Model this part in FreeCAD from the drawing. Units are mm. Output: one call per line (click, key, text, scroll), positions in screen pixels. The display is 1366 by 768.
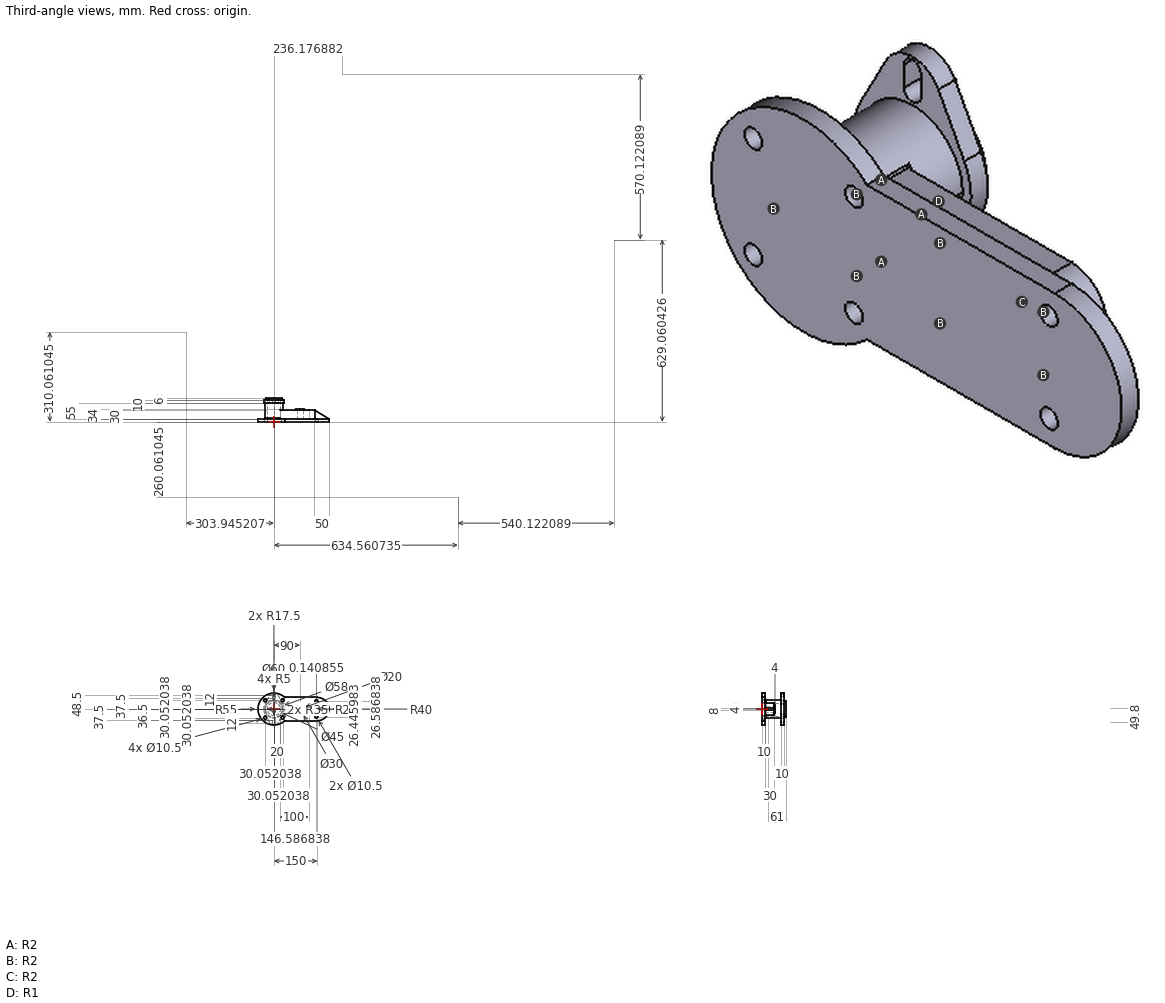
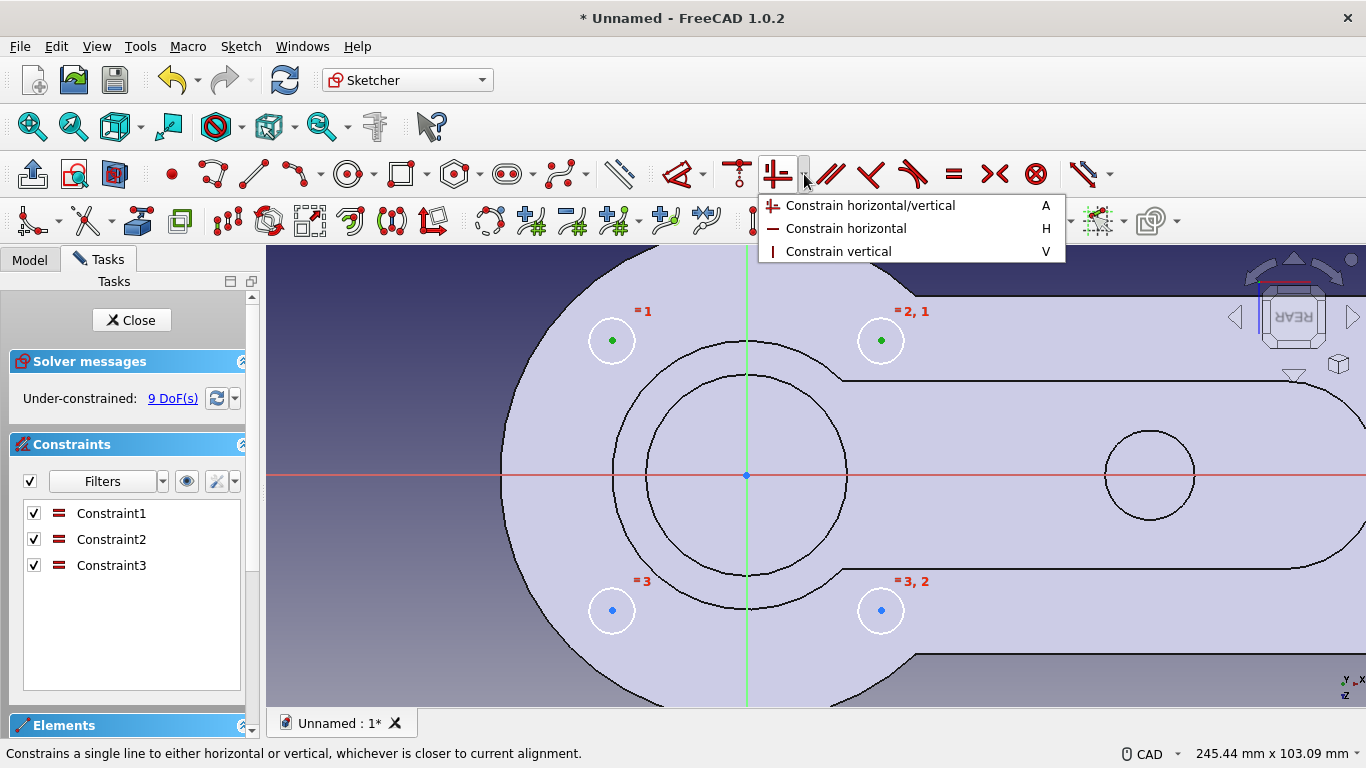
click(912, 228)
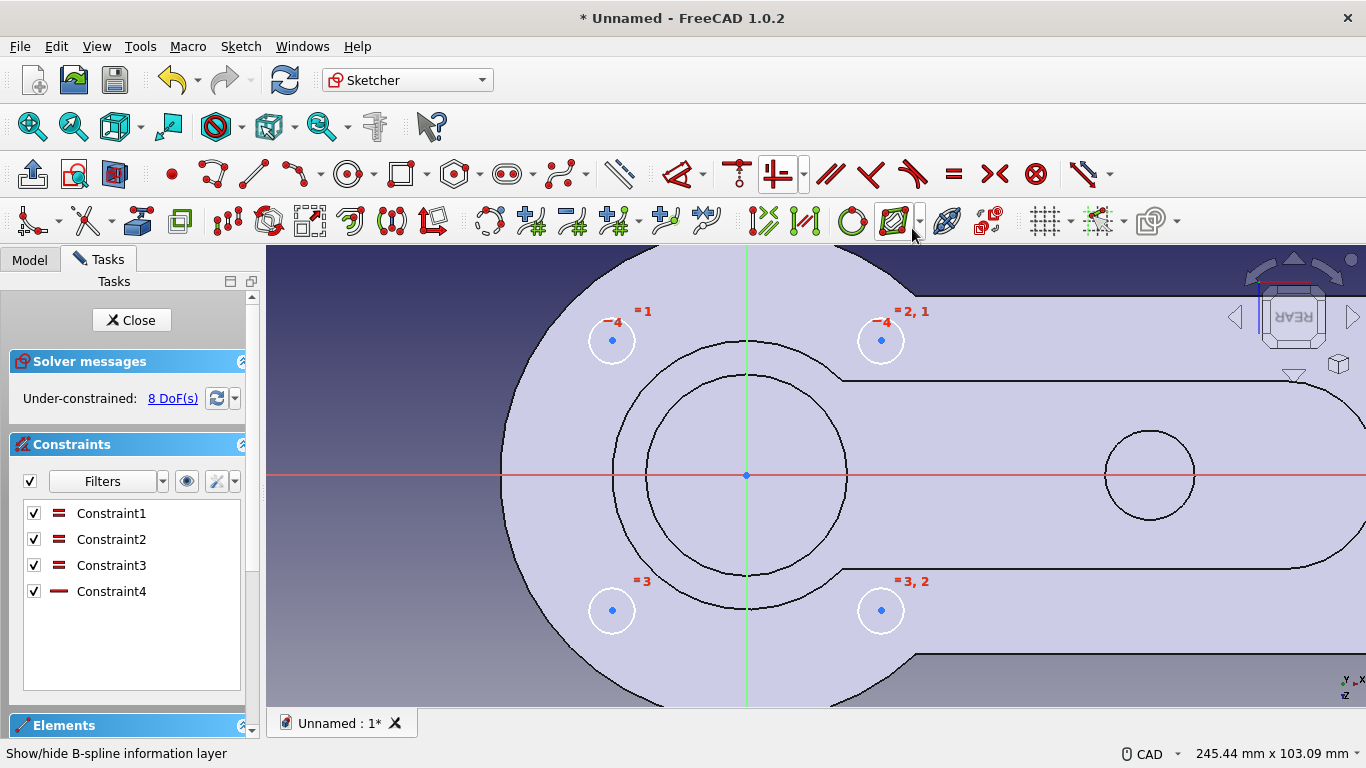
click(881, 341)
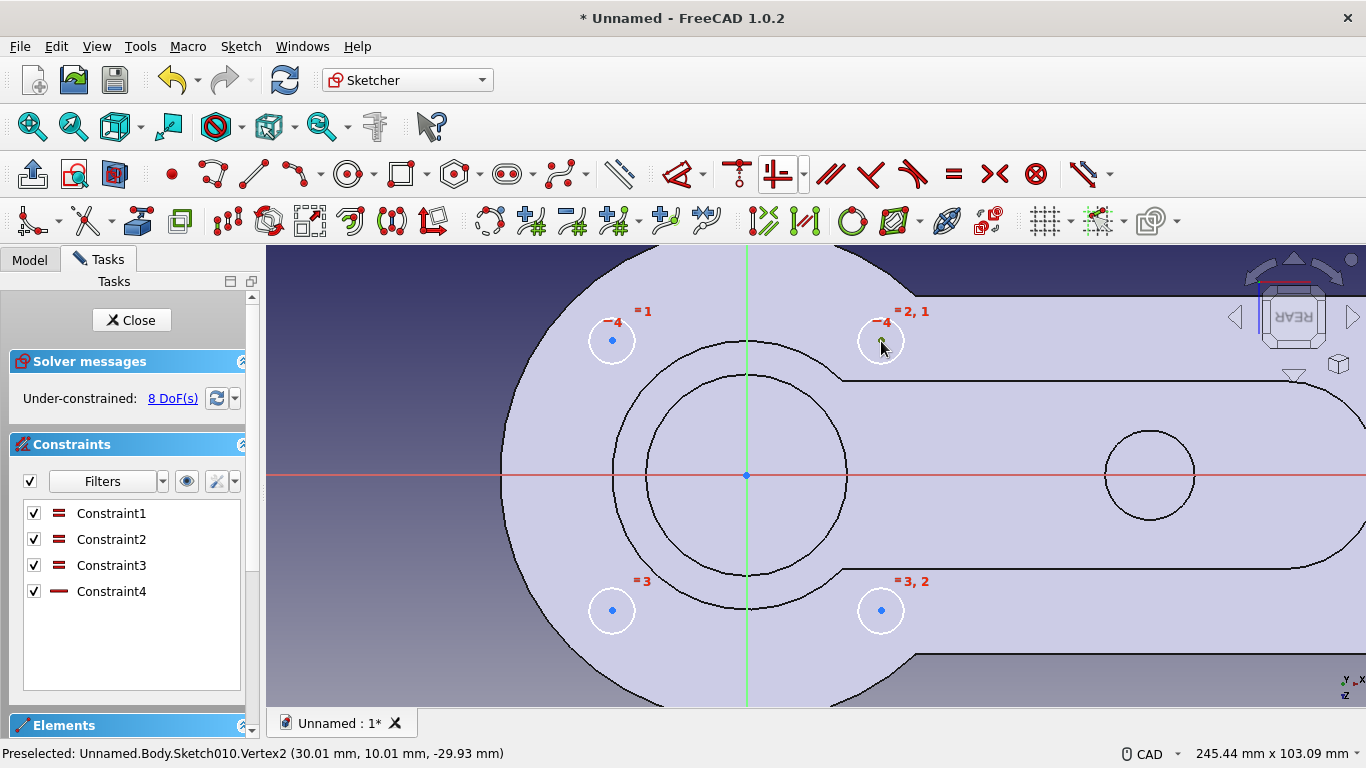
click(881, 611)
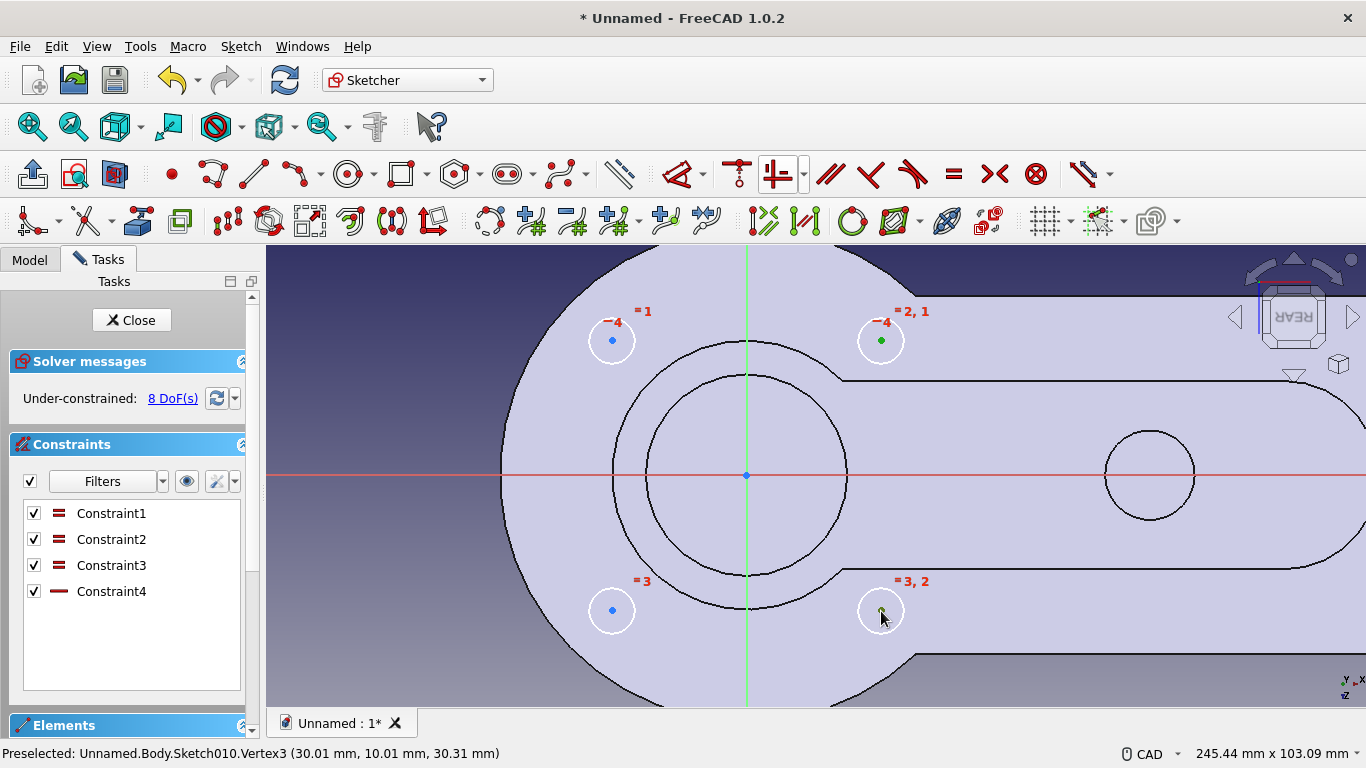
key(v)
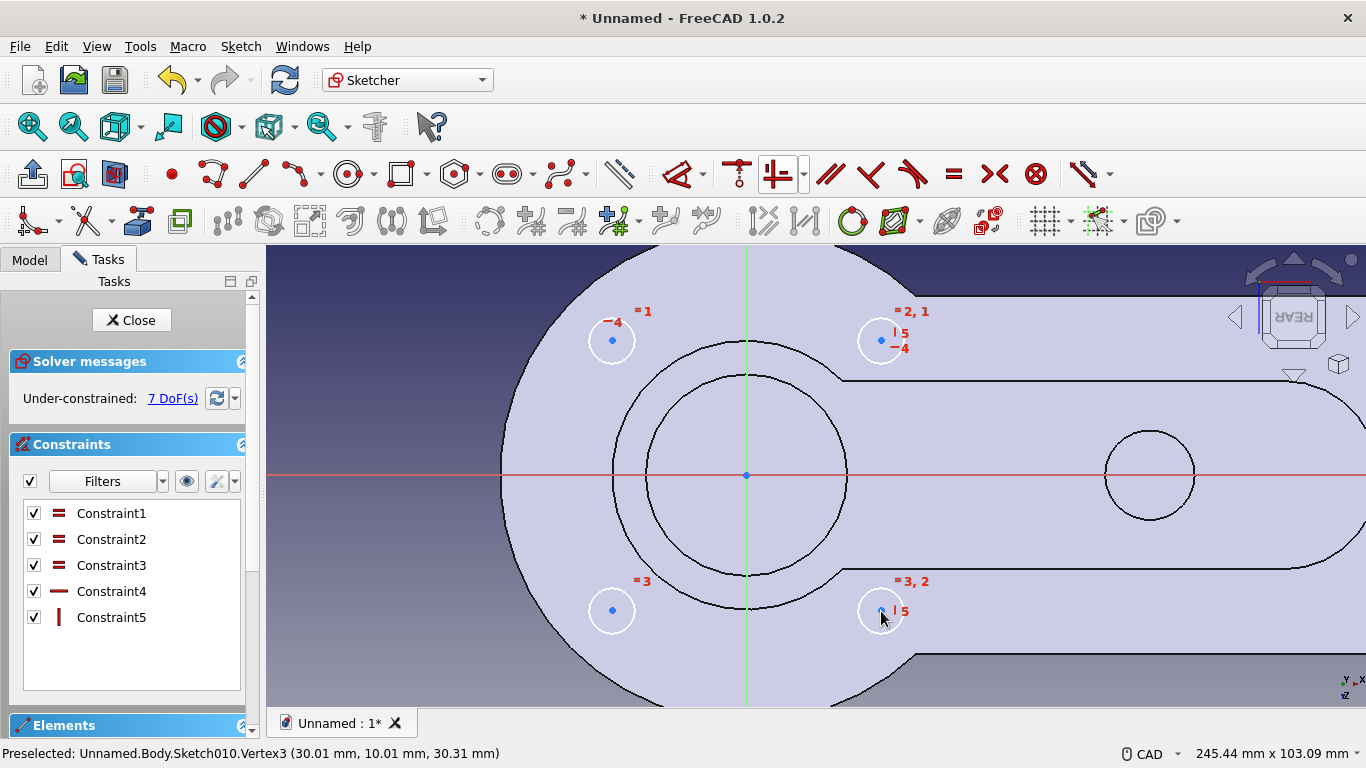
click(612, 341)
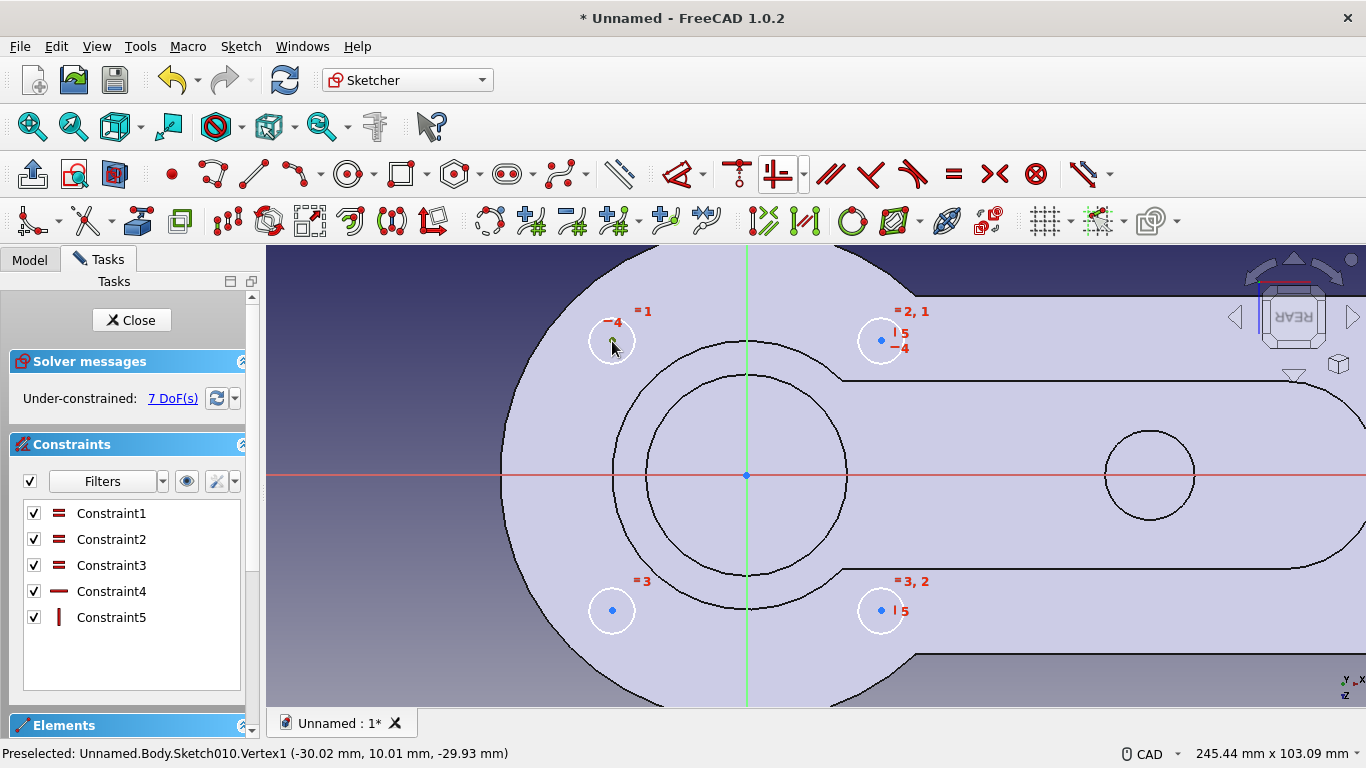
click(612, 611)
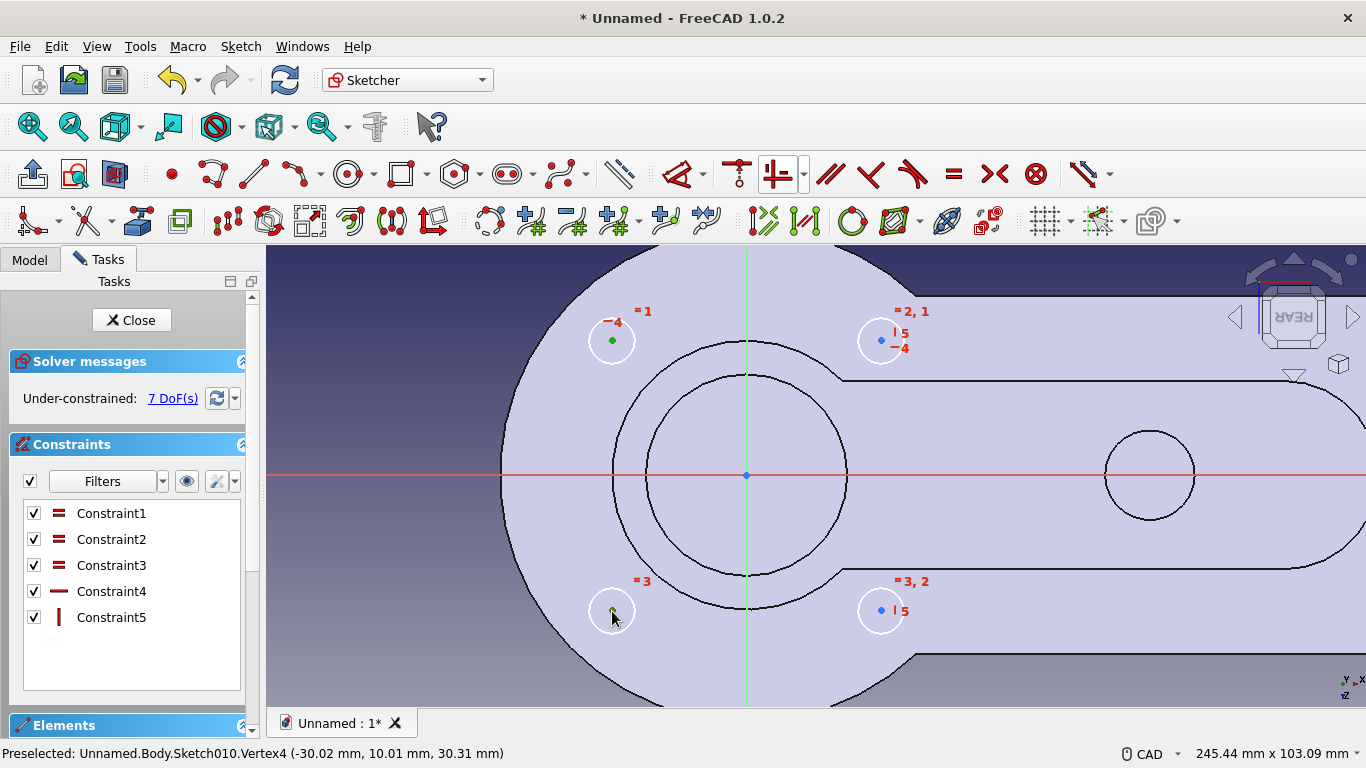
key(v)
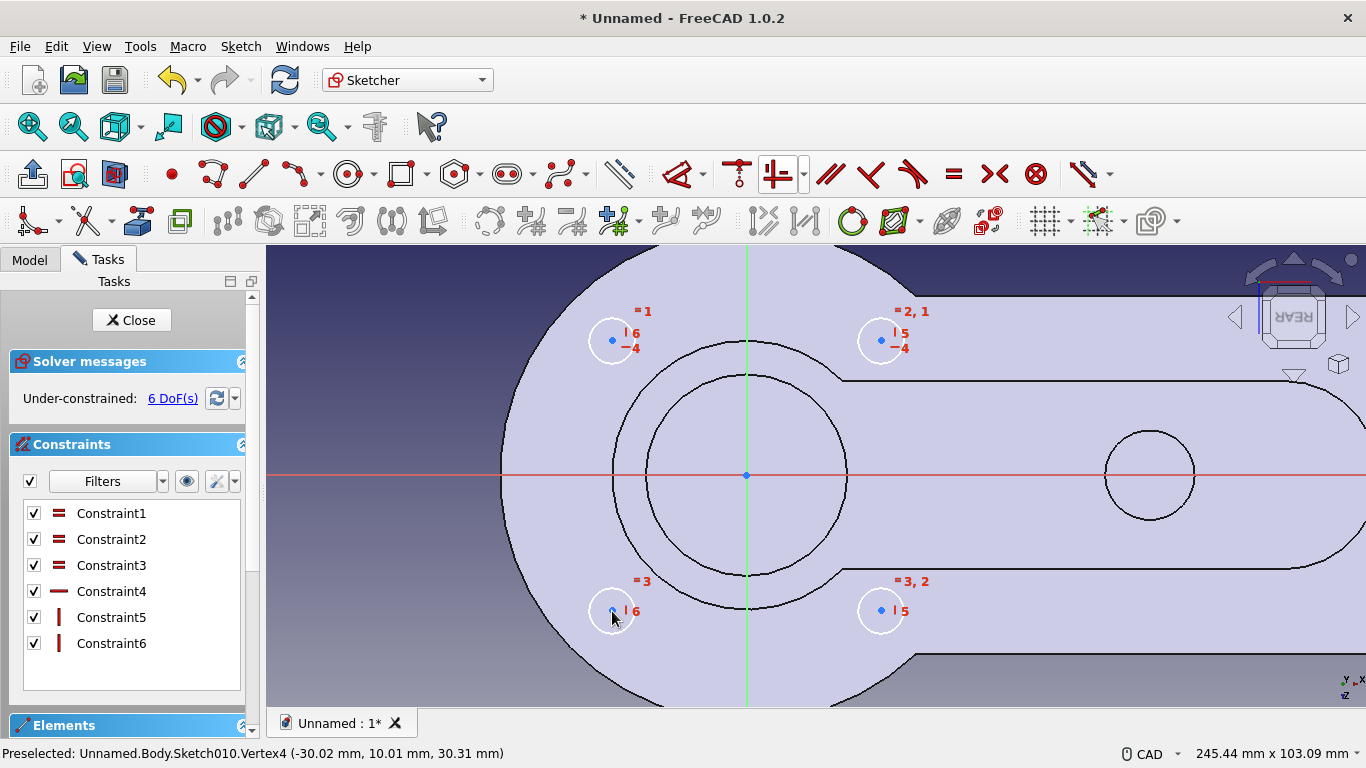
click(881, 611)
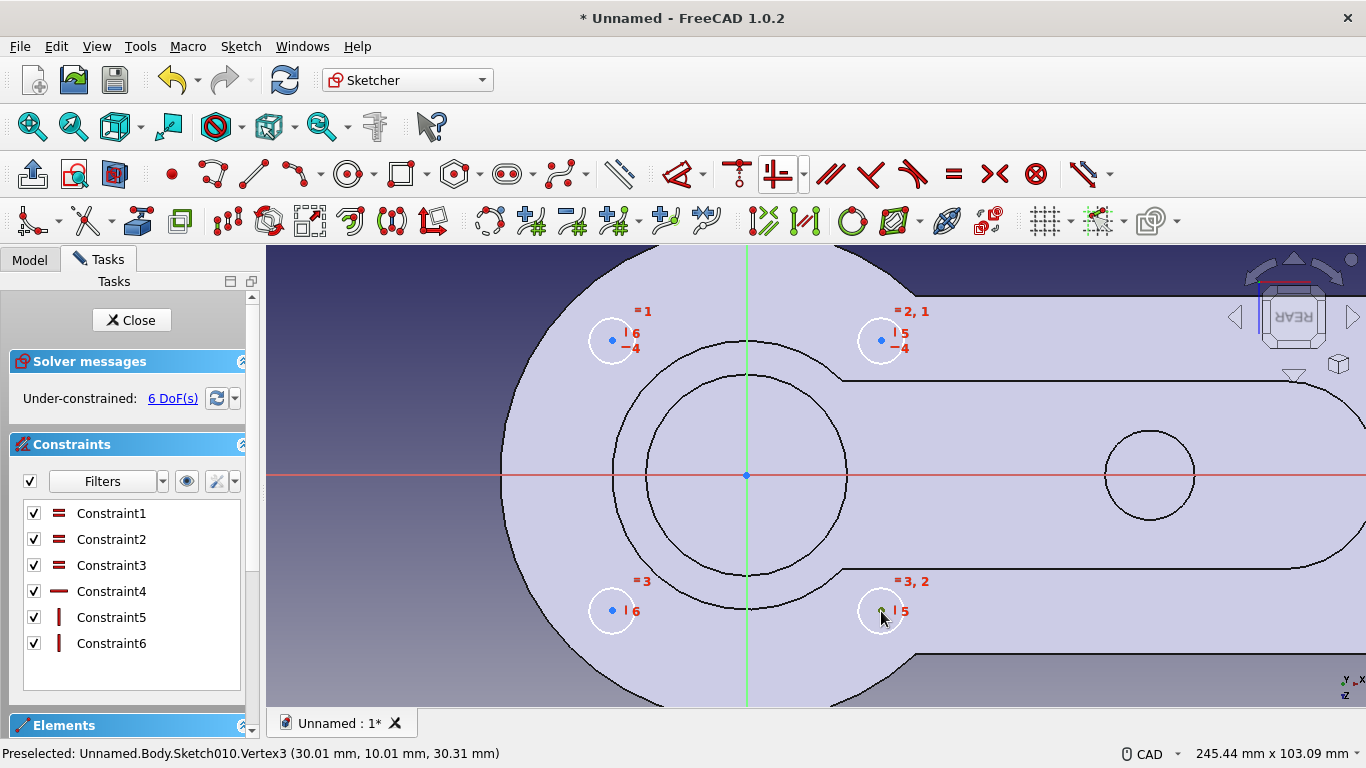
click(612, 611)